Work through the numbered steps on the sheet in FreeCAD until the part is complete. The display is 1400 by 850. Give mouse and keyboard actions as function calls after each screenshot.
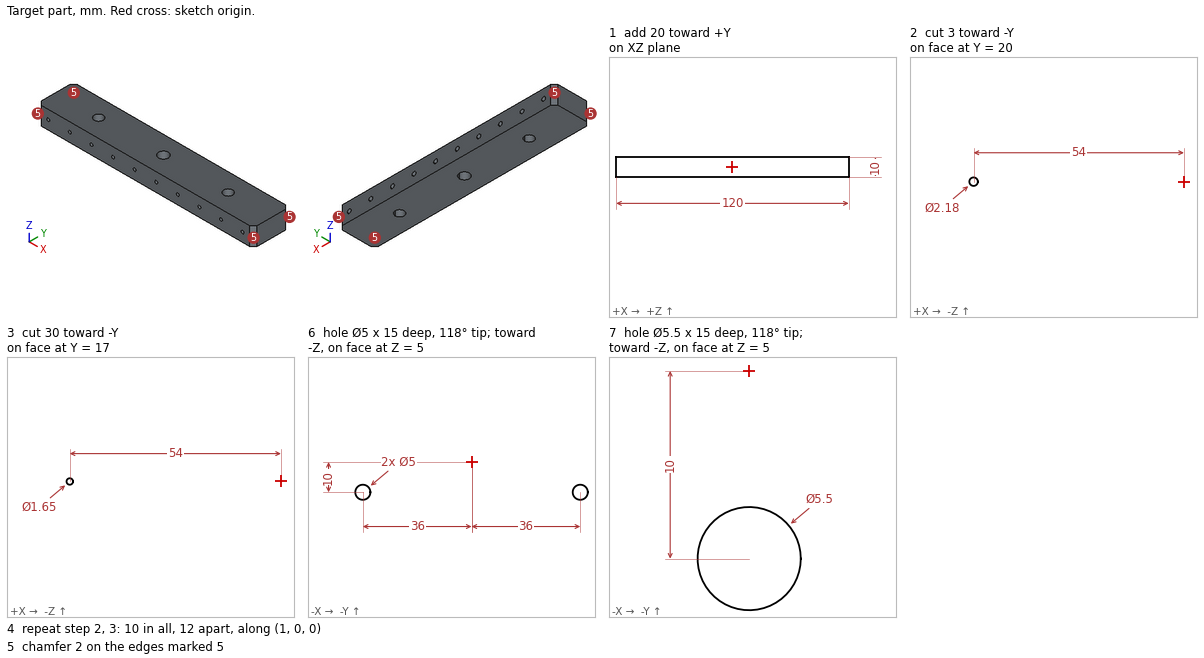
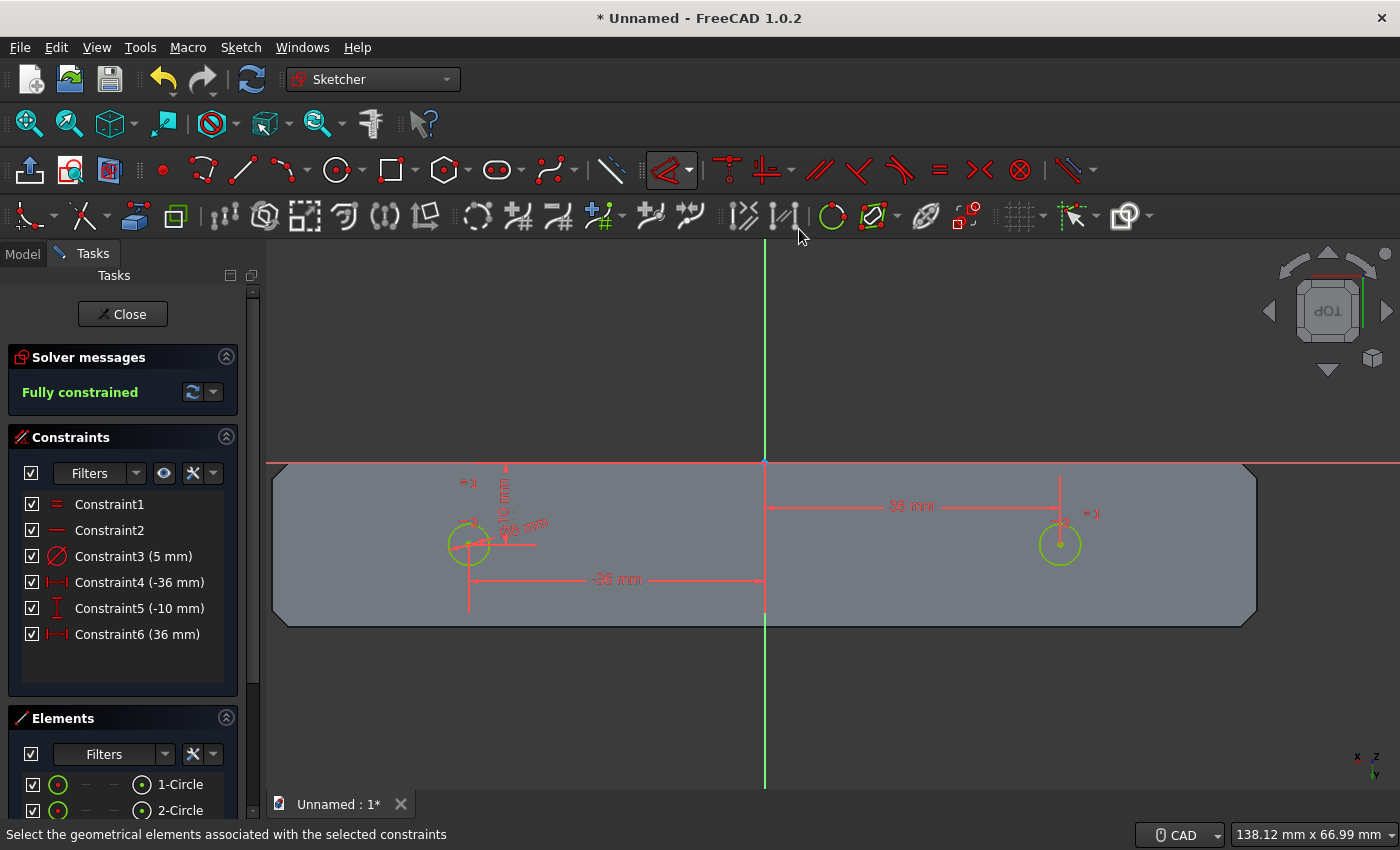
click(123, 314)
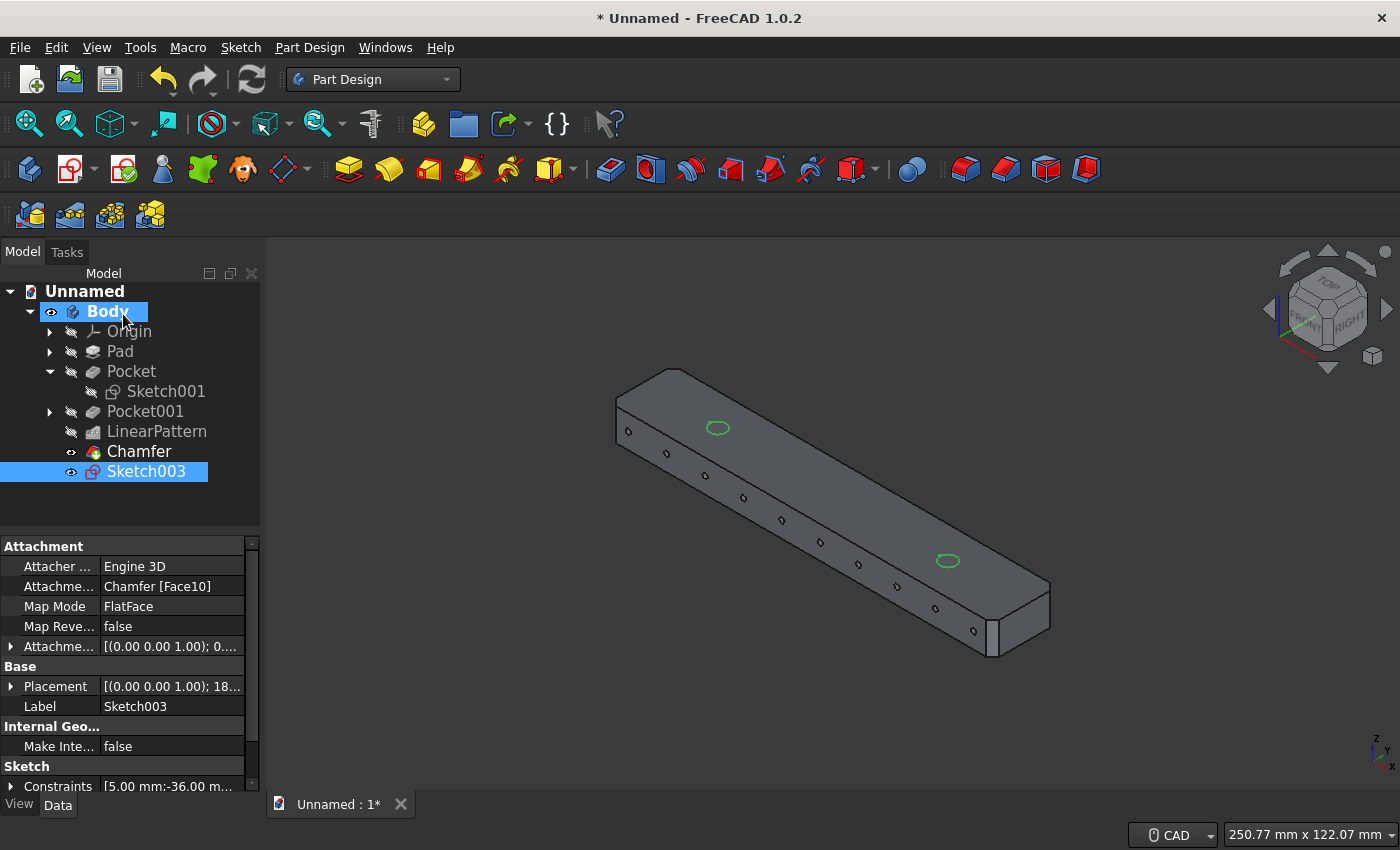
click(652, 170)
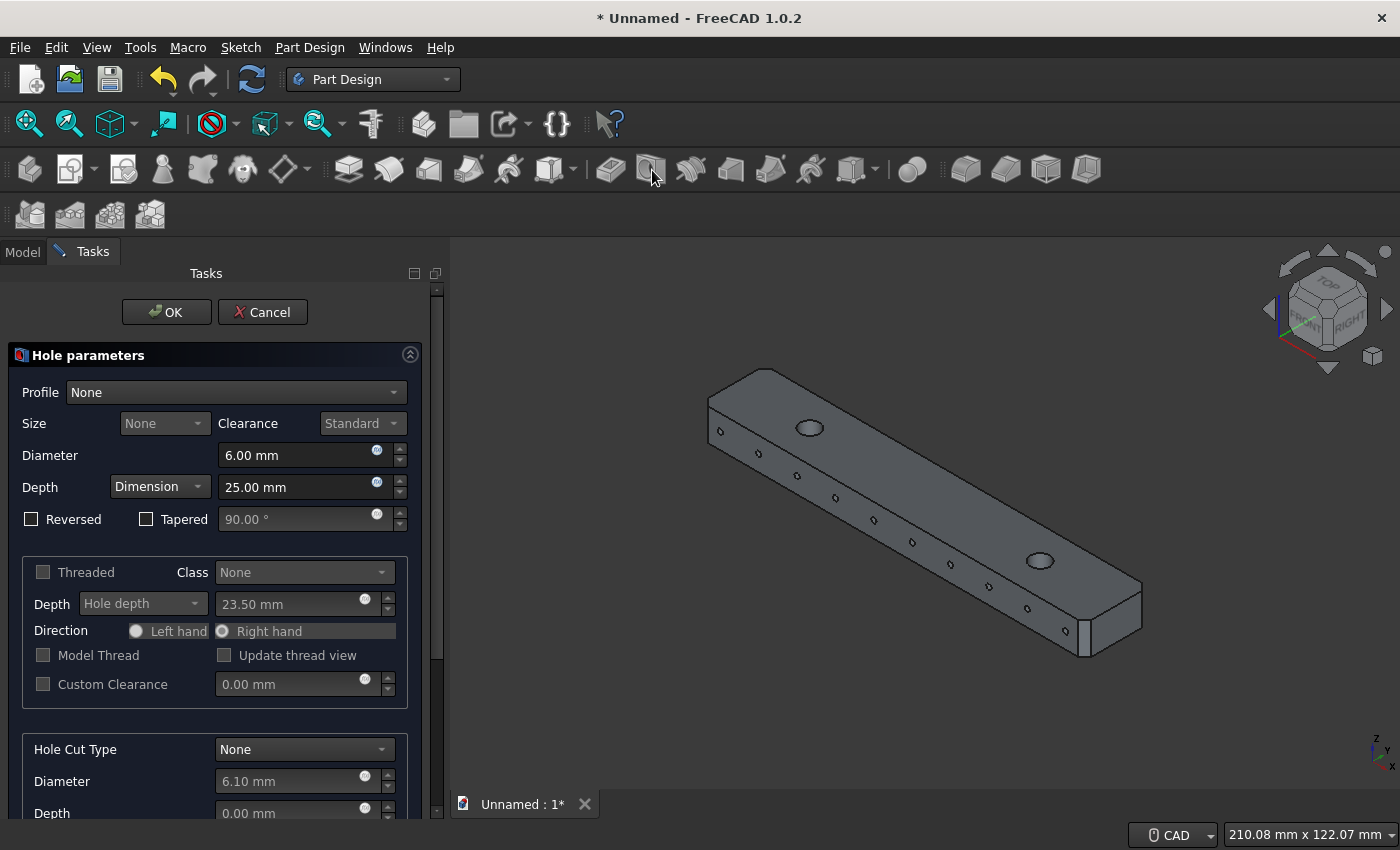
triple_click(305, 455)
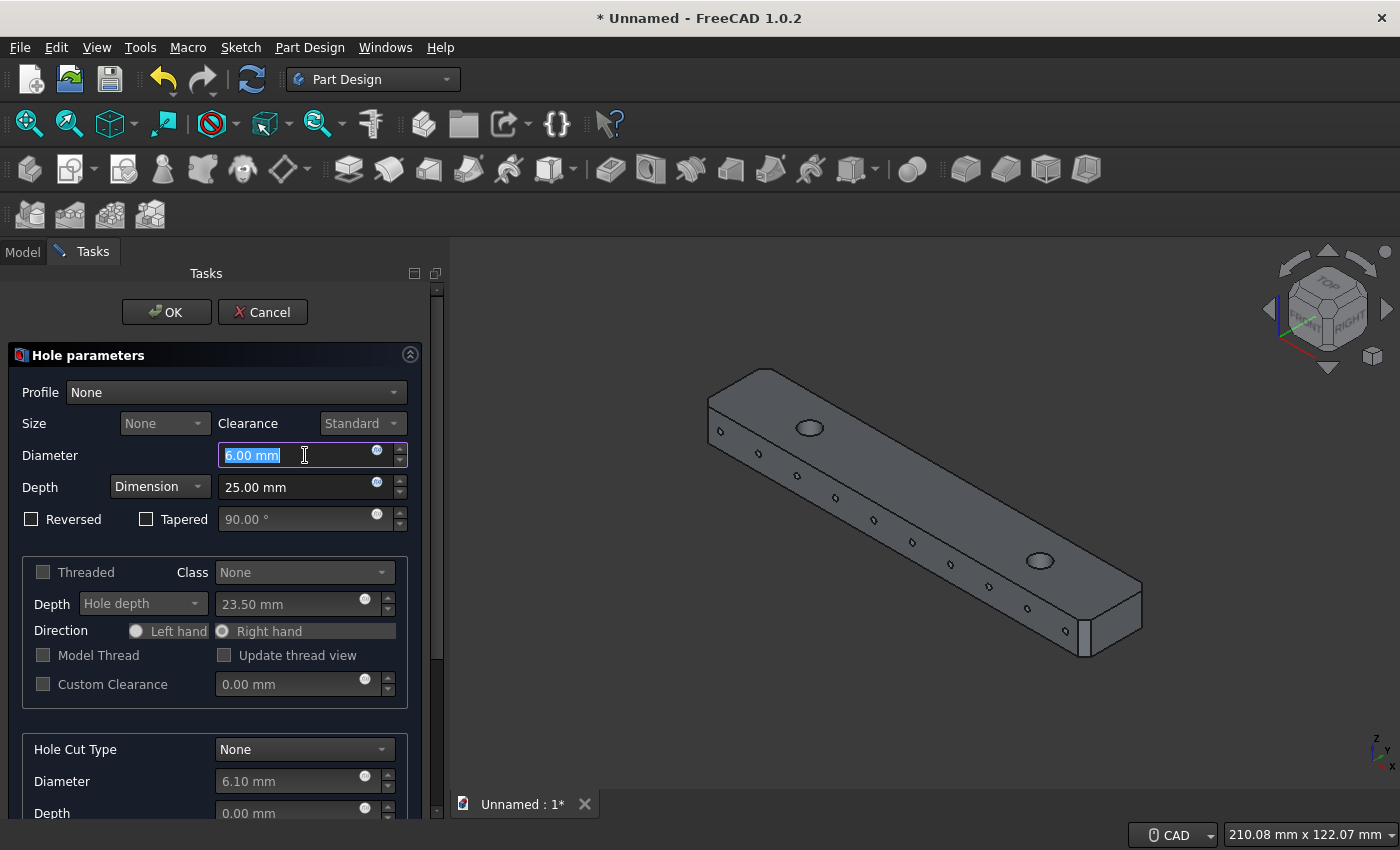
text(5)
key(Tab)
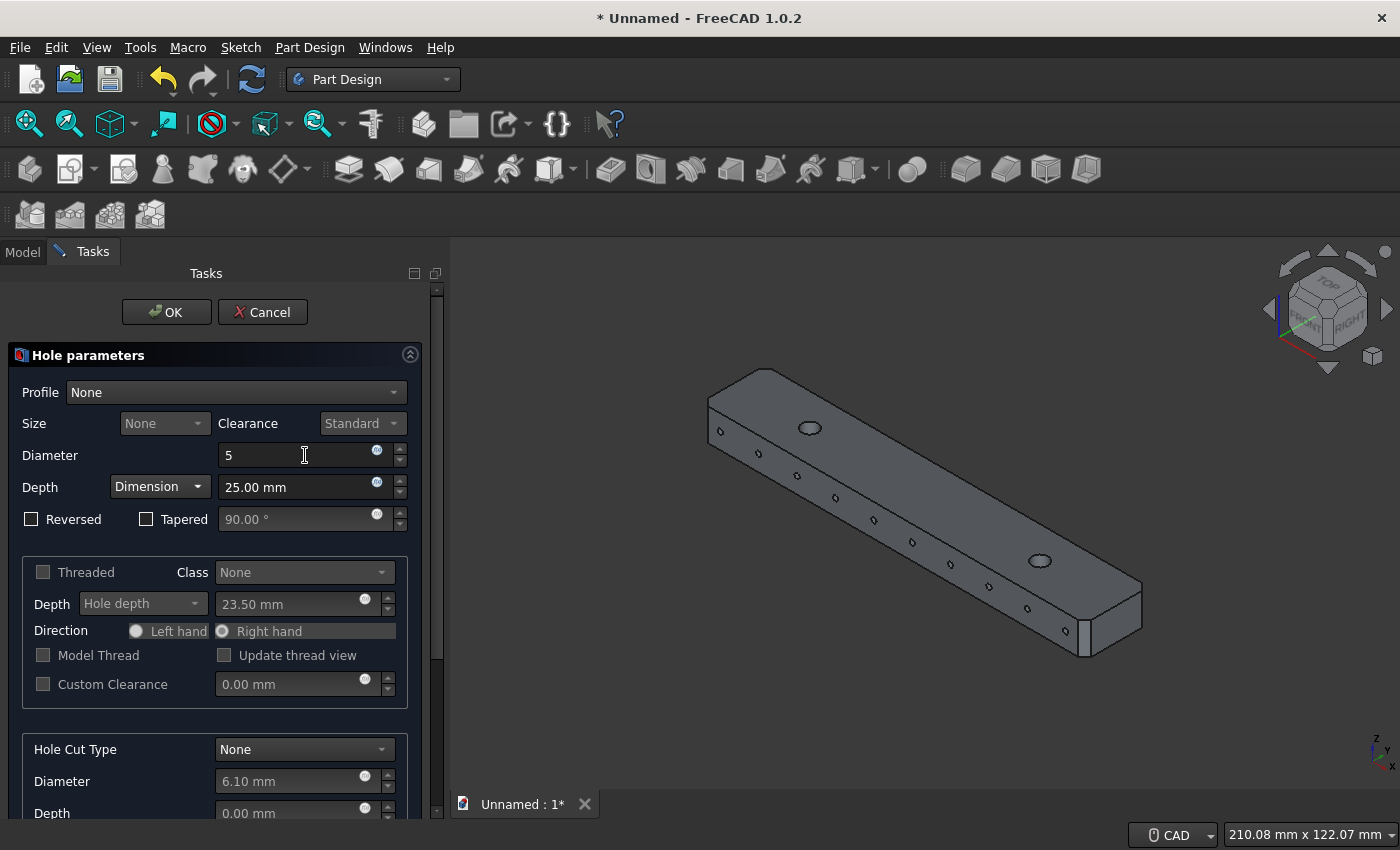
triple_click(305, 487)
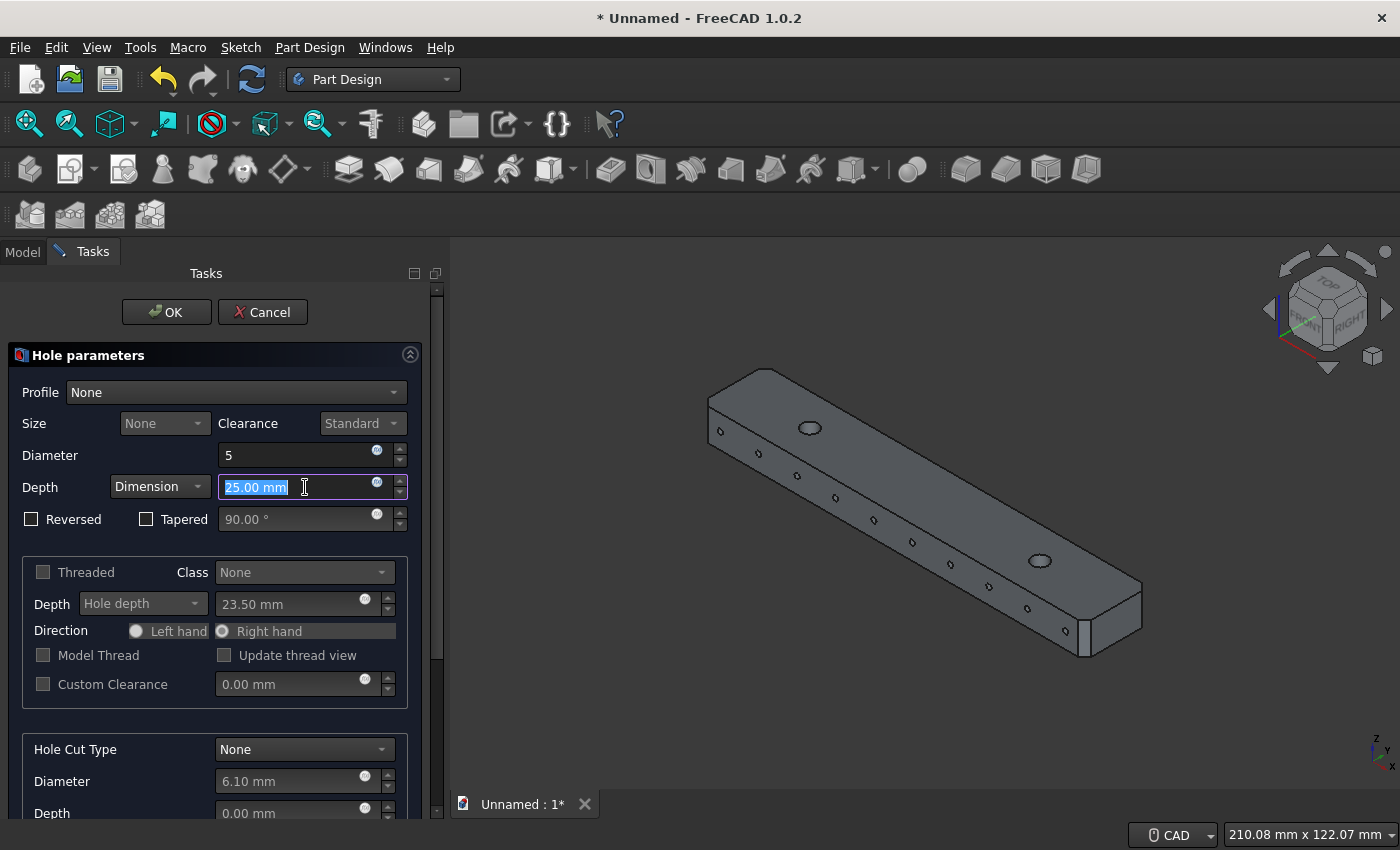
text(15)
key(Tab)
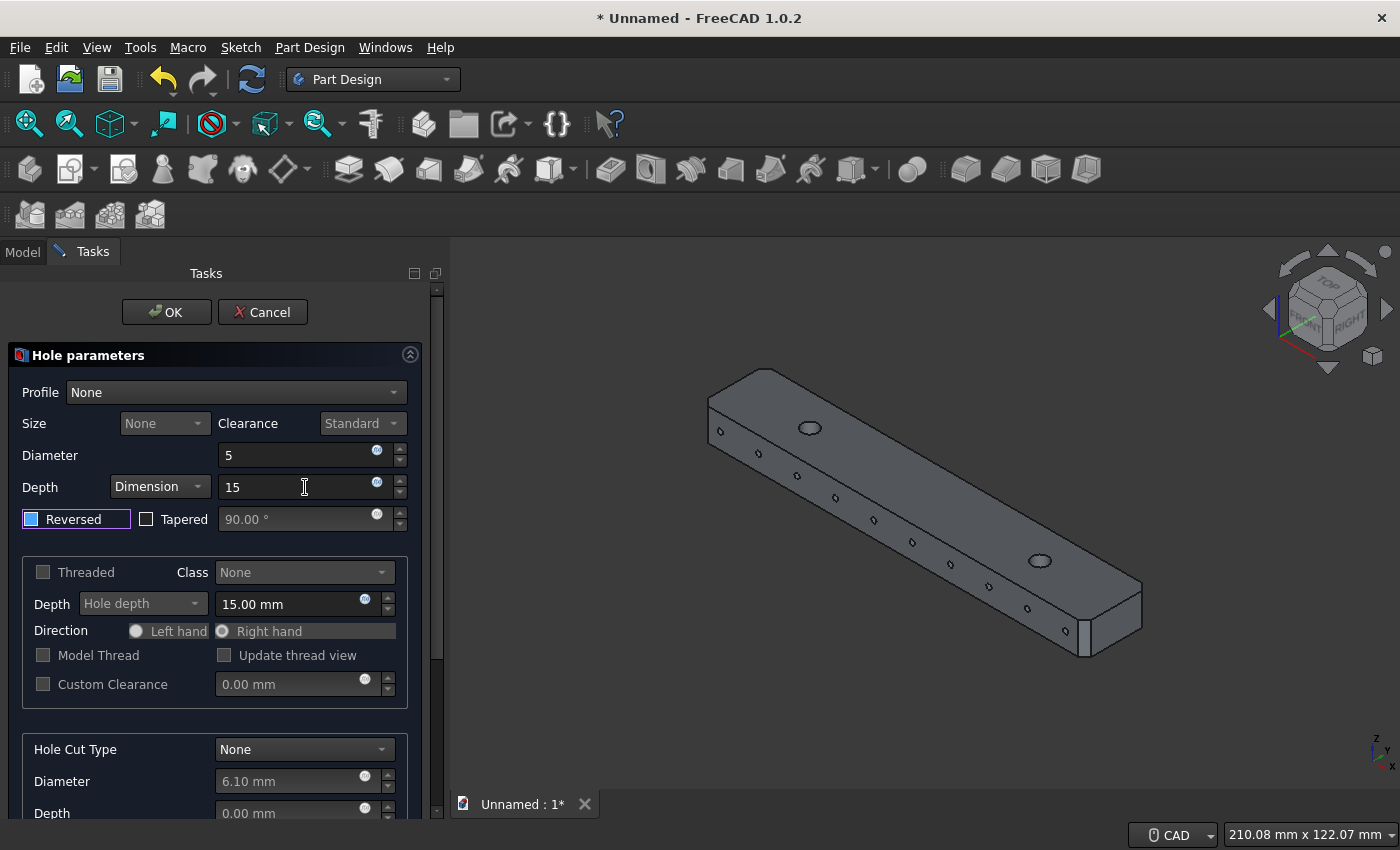
click(167, 312)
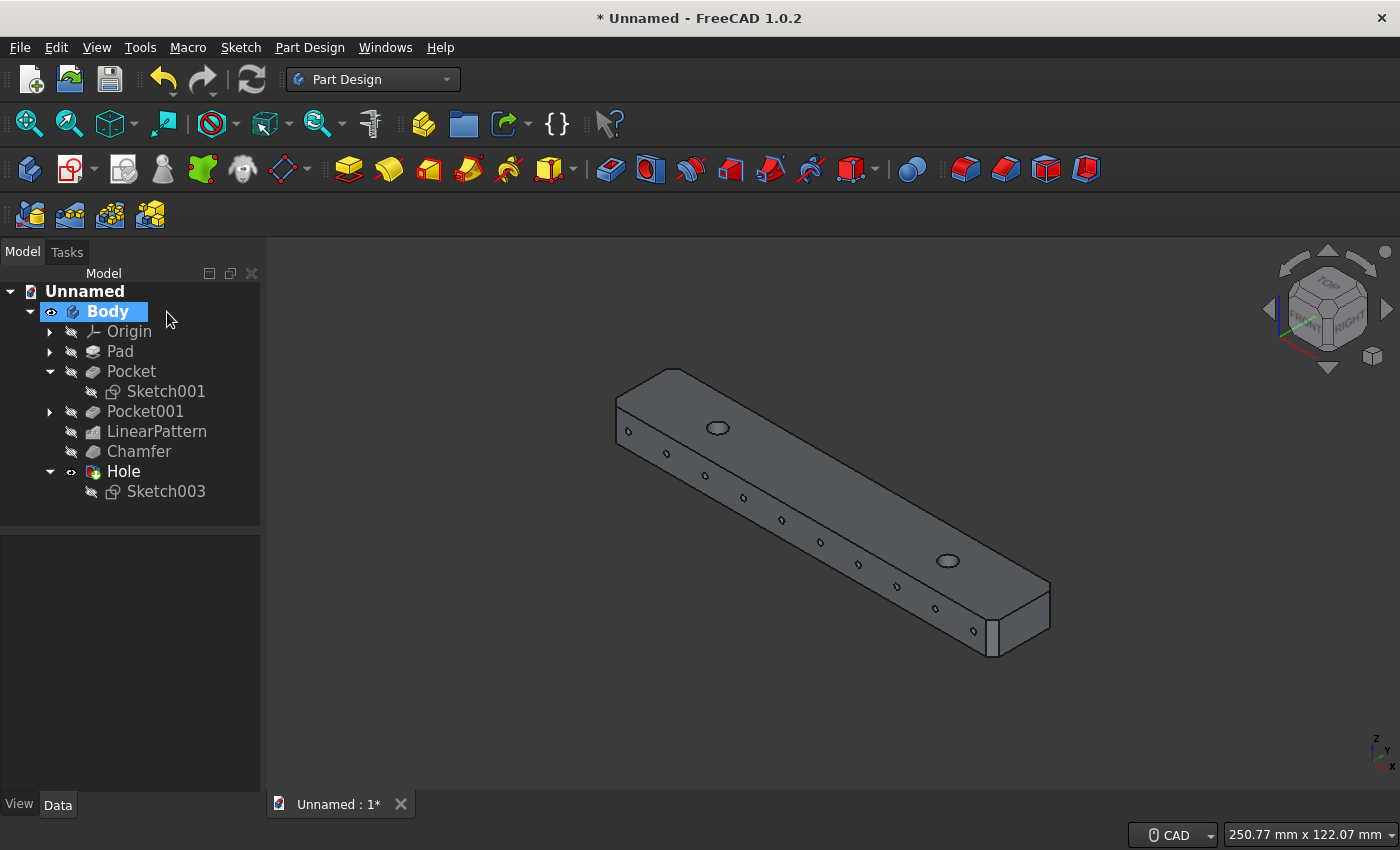
click(888, 525)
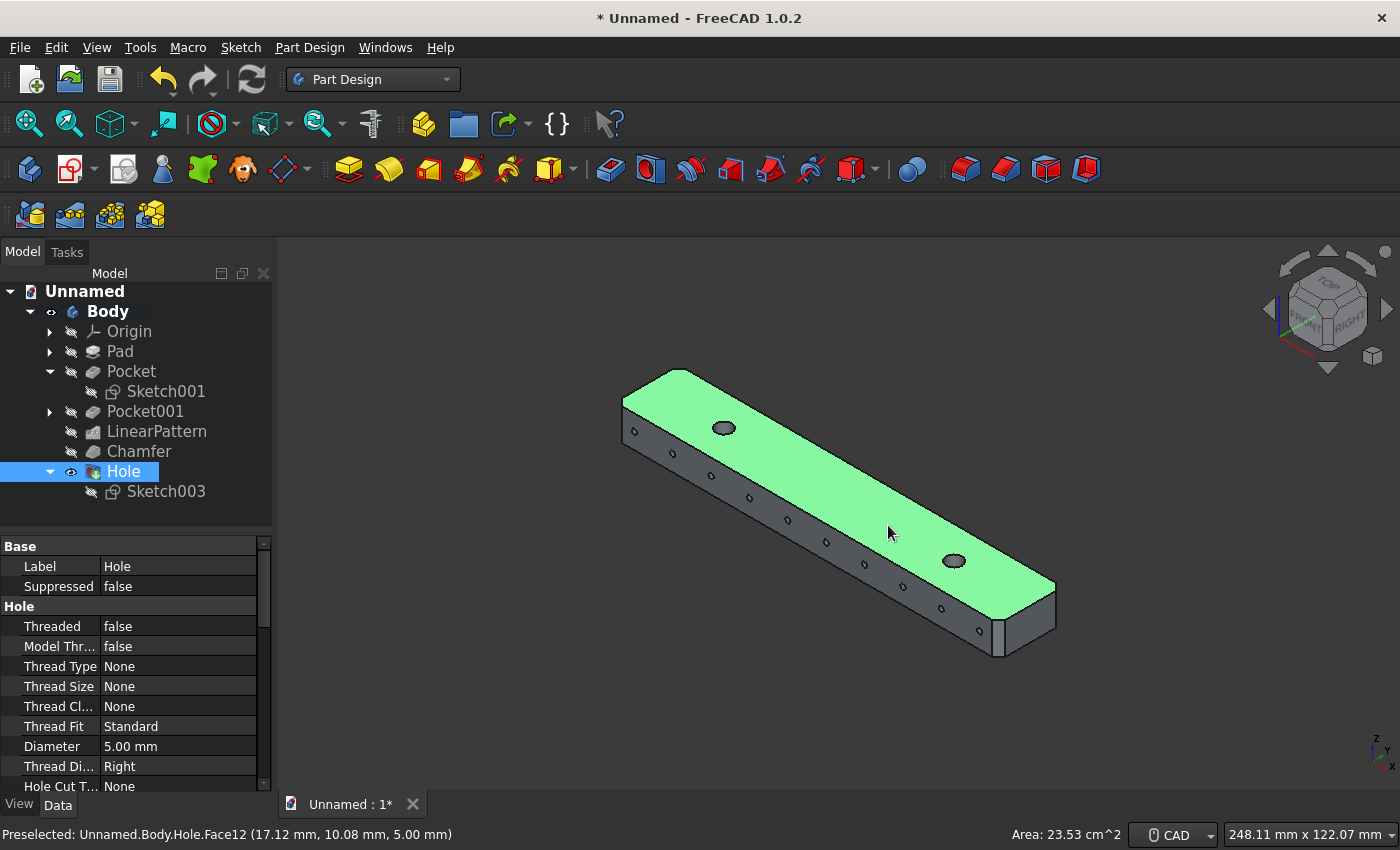
click(70, 170)